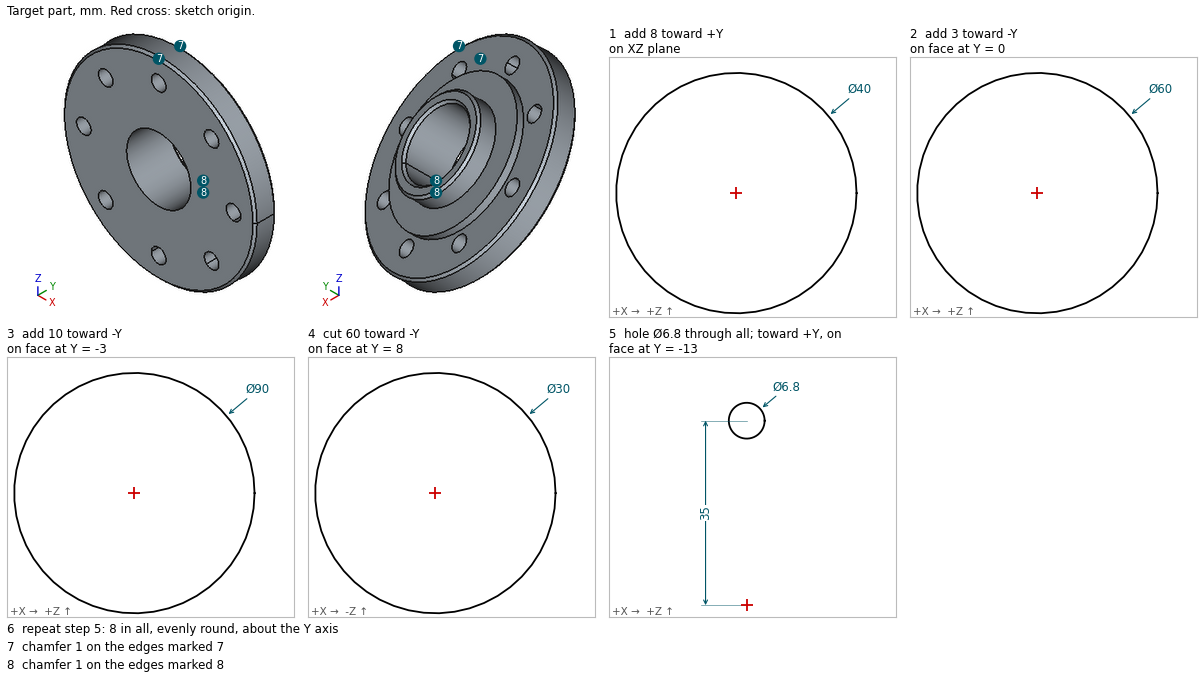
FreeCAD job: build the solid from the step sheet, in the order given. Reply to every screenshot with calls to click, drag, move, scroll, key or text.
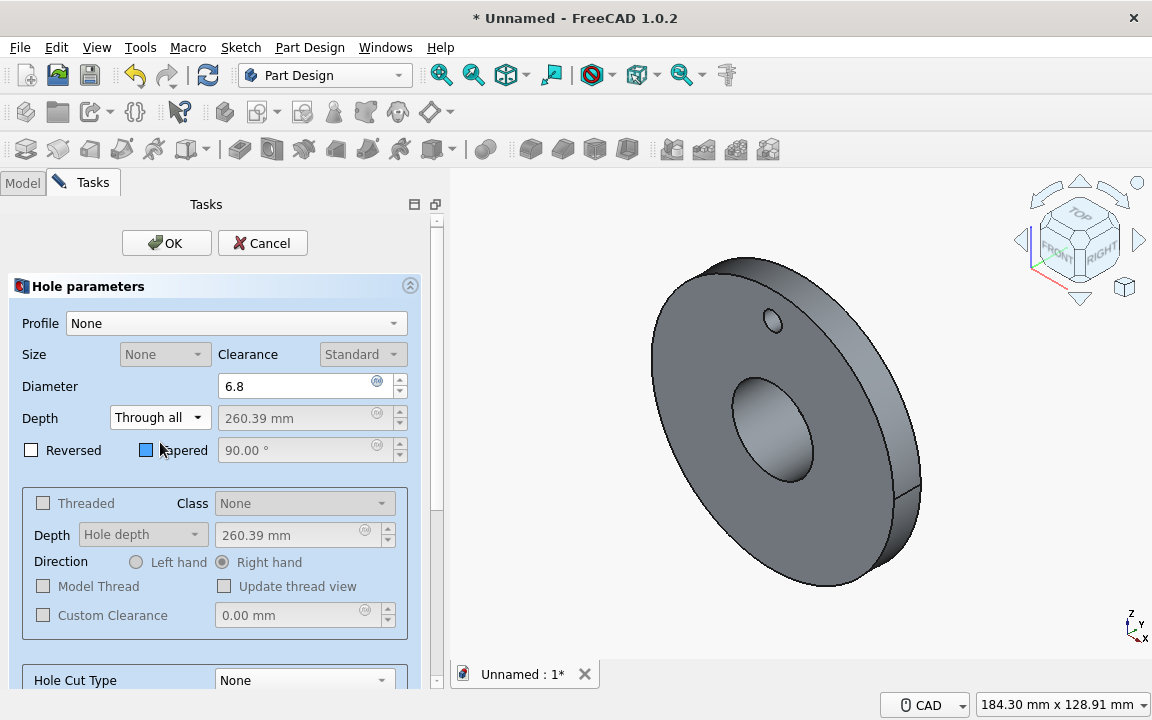
click(167, 243)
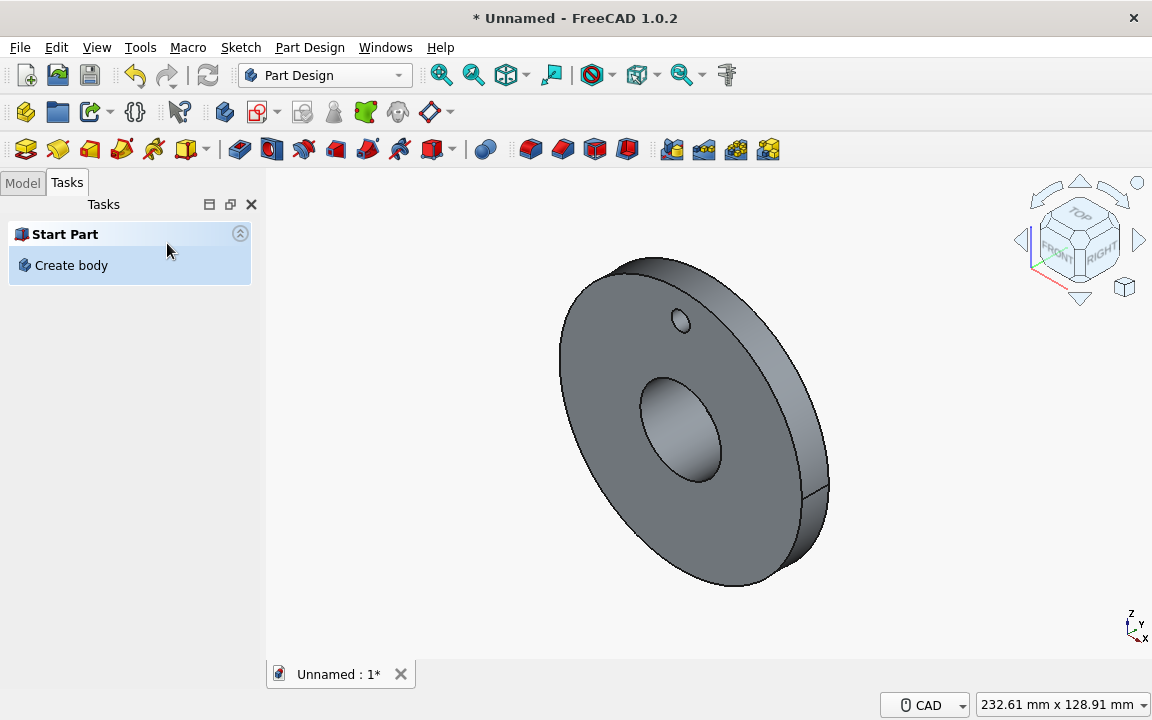
click(23, 182)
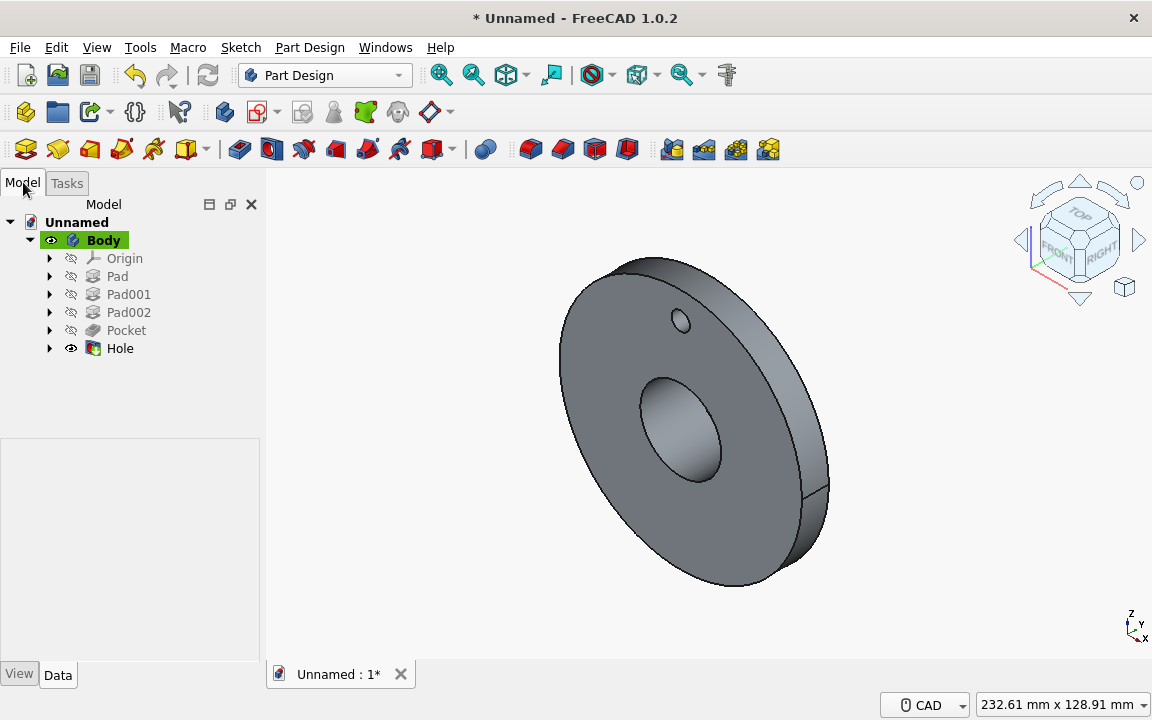
click(116, 348)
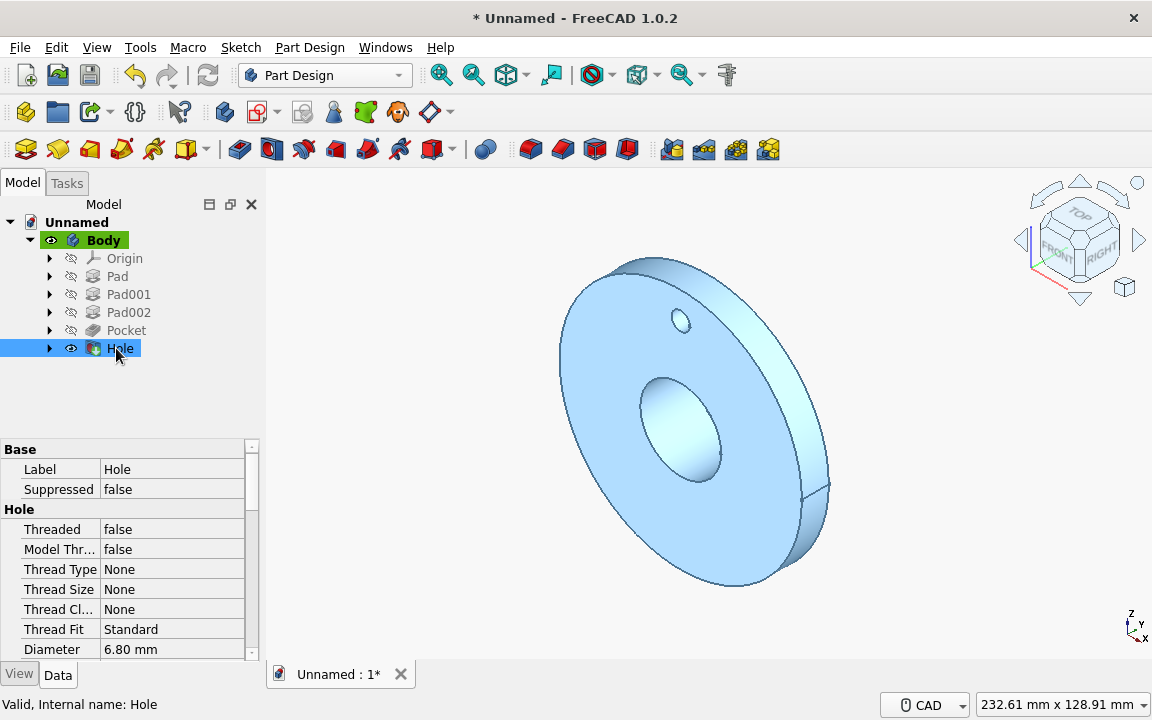
click(736, 150)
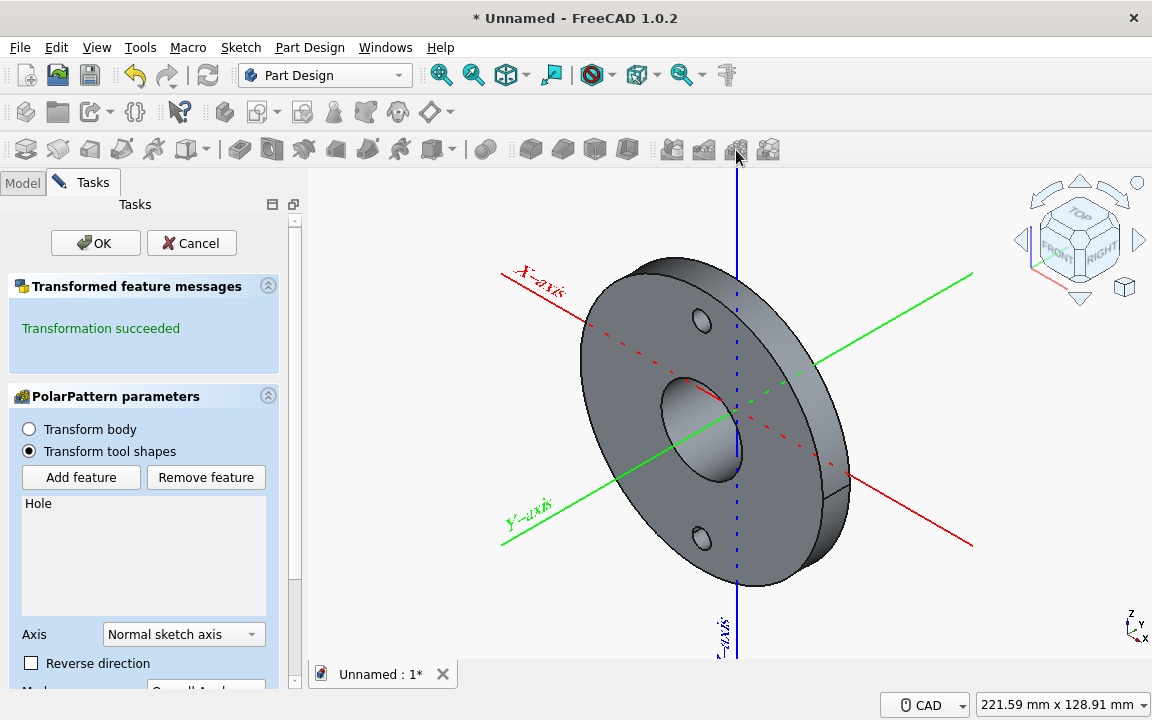
click(184, 634)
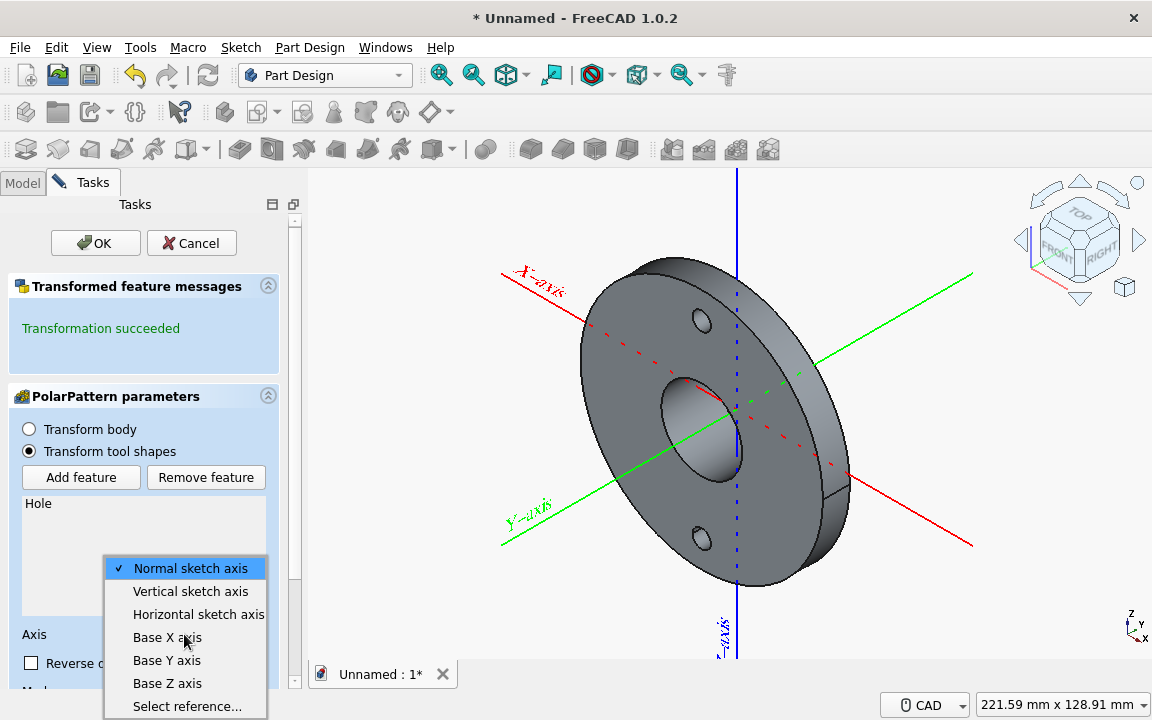
click(184, 660)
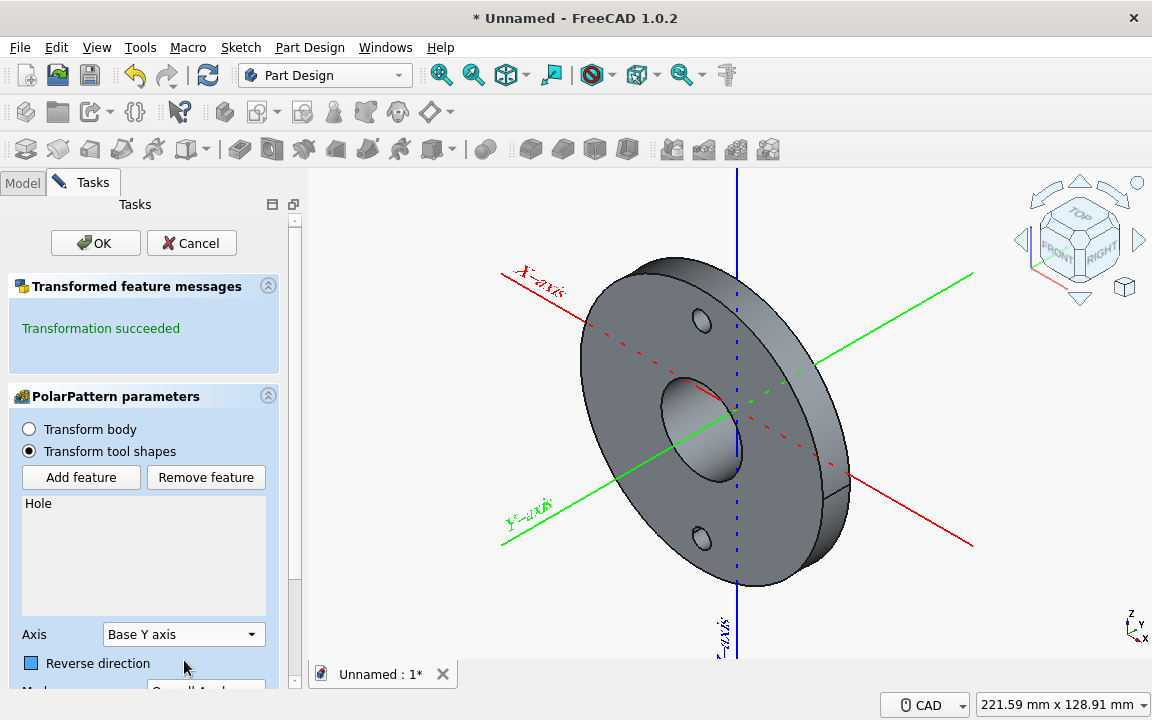
scroll(295, 451, down, 3)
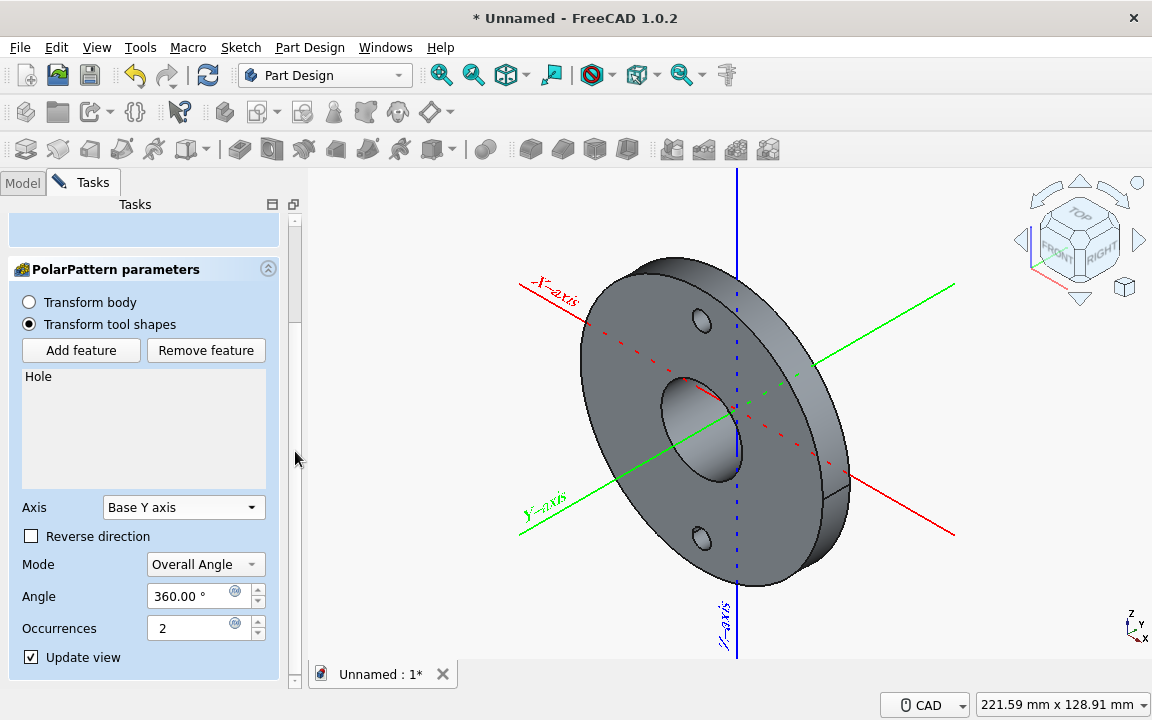
triple_click(198, 628)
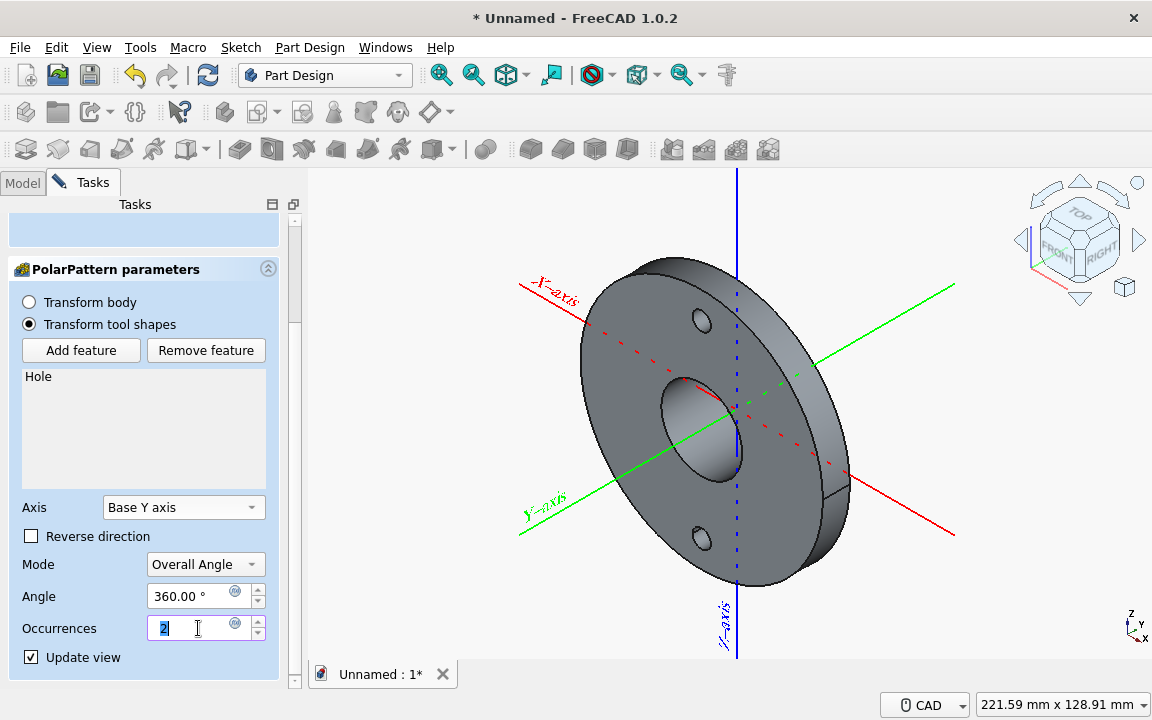
text(8)
key(Tab)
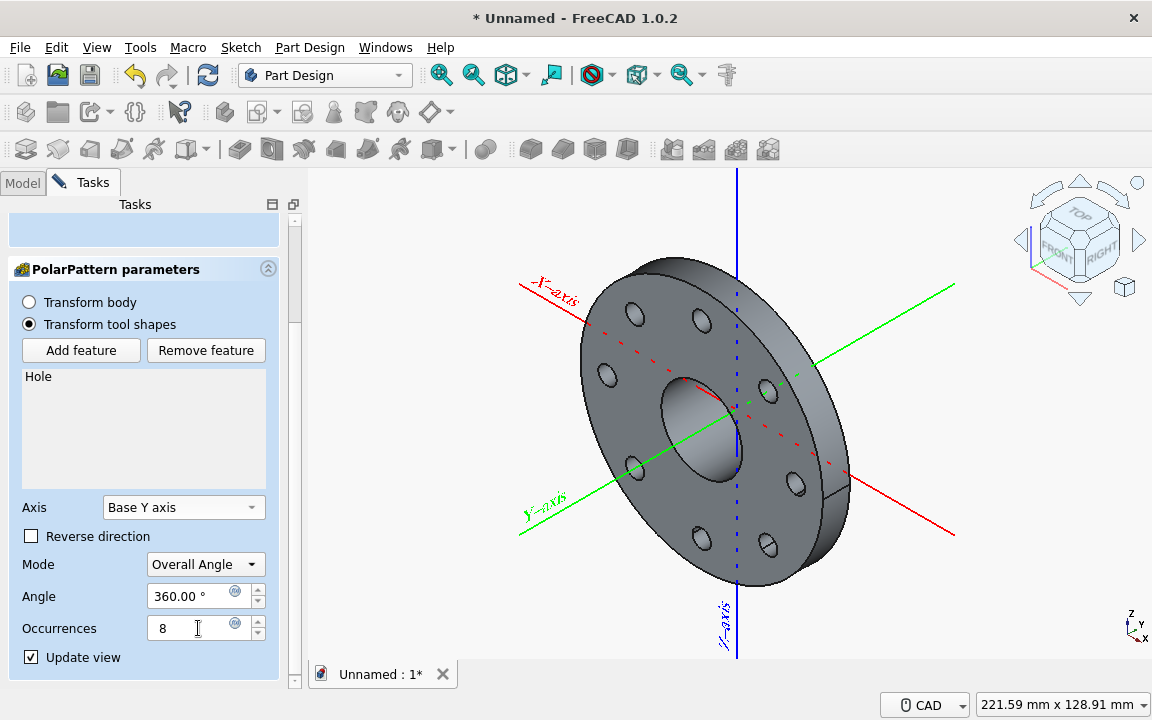
scroll(295, 451, up, 3)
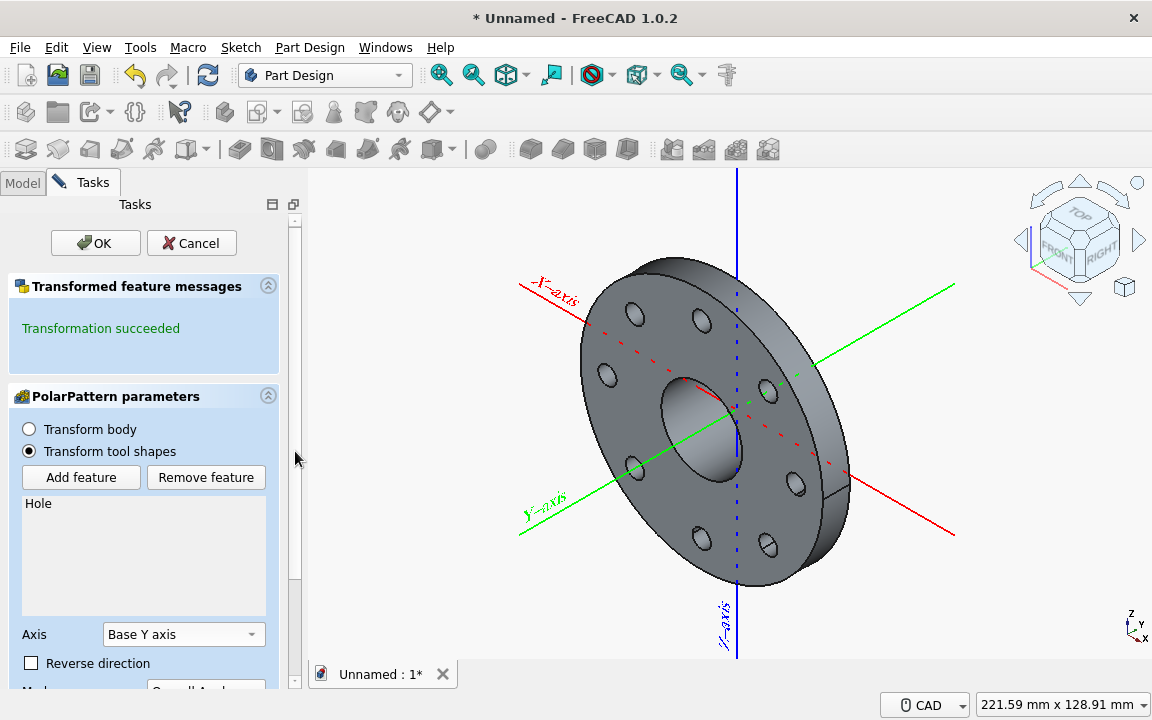
click(96, 243)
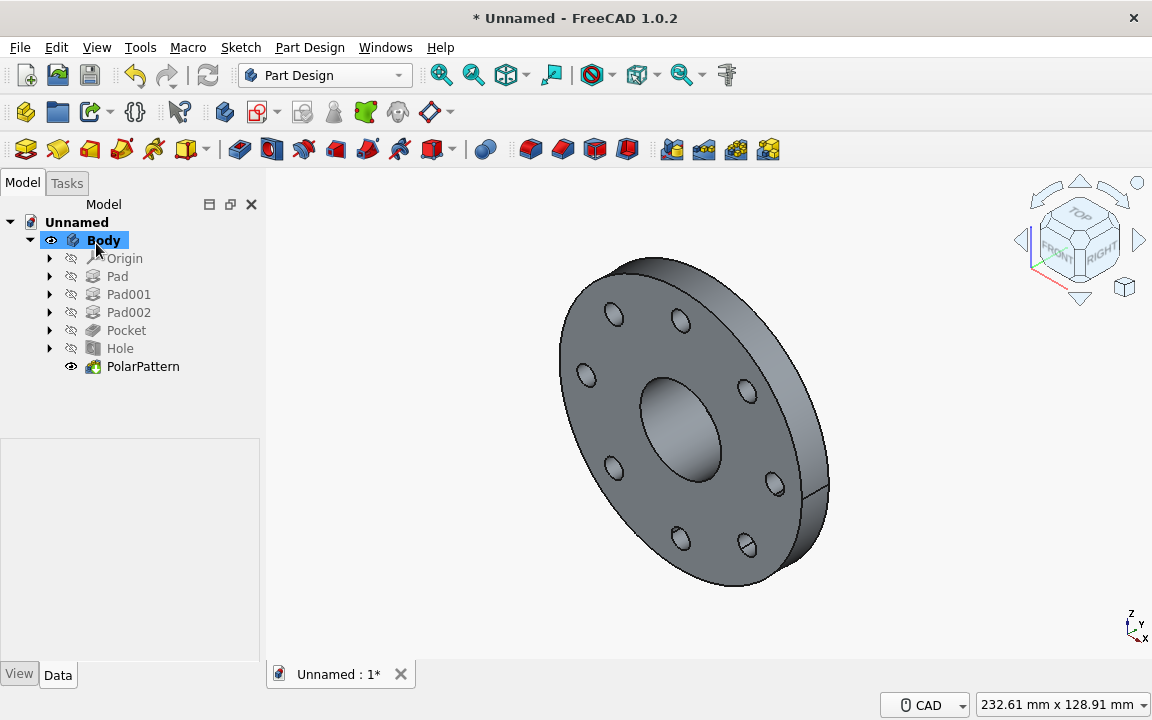
click(643, 274)